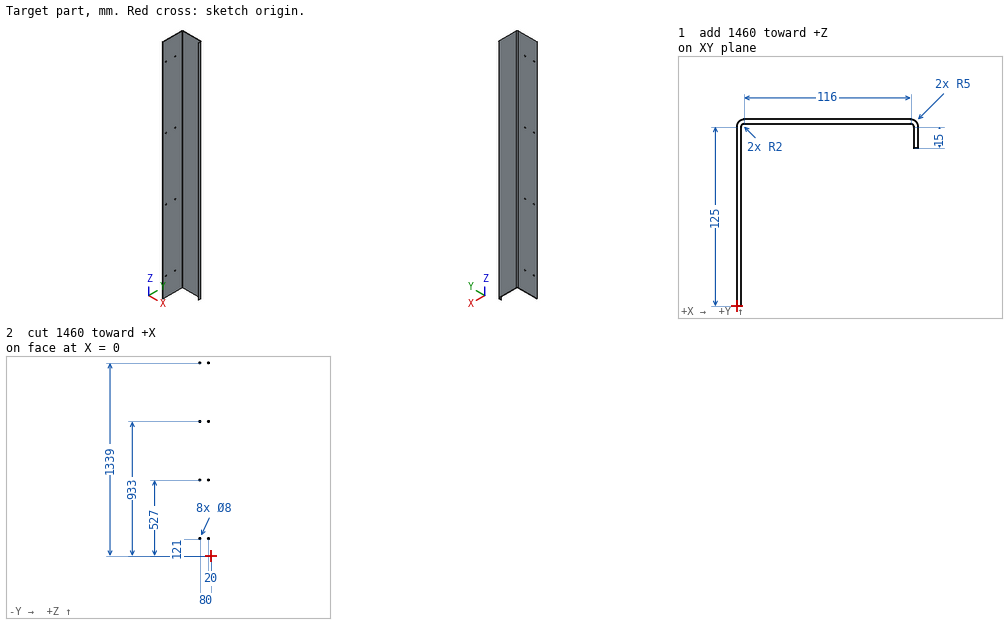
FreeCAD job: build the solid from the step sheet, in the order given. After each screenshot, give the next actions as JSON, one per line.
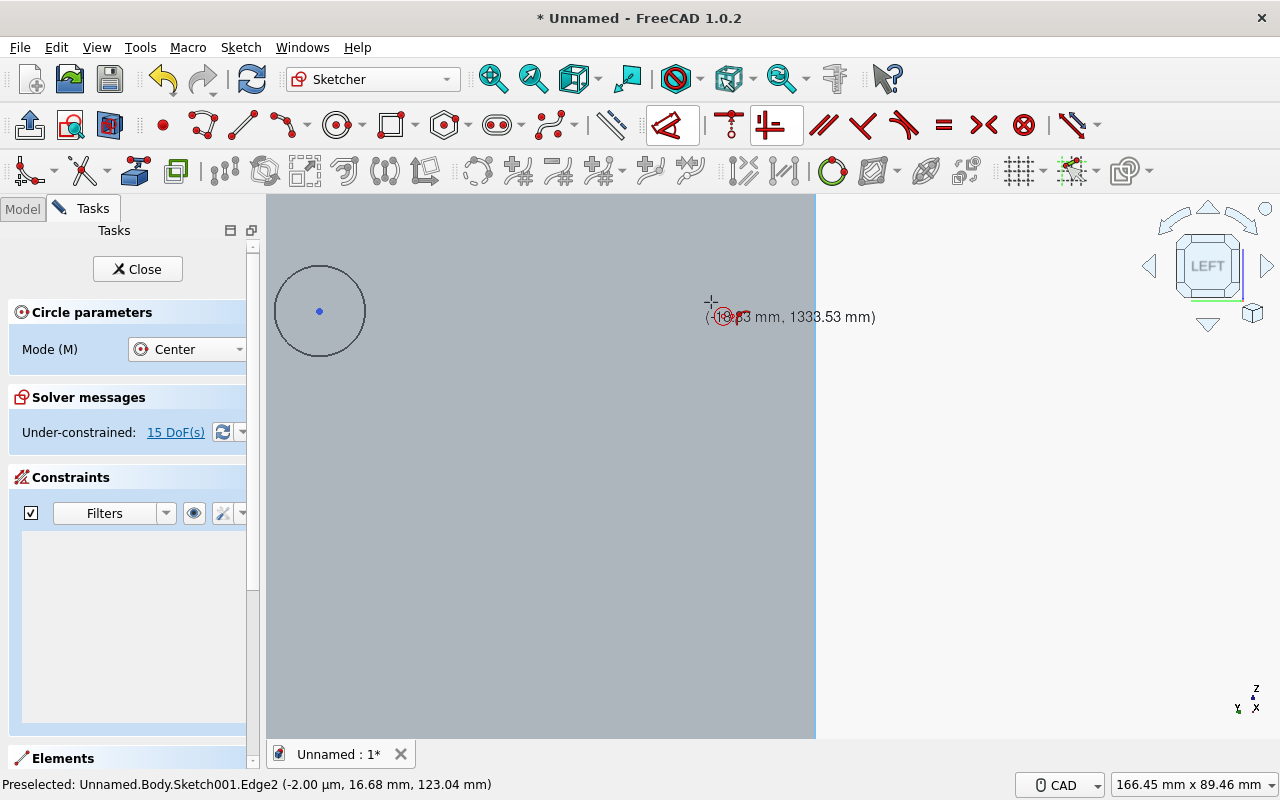
{"action": "scroll", "coordinate": [712, 263], "scroll_direction": "down", "scroll_amount": 15}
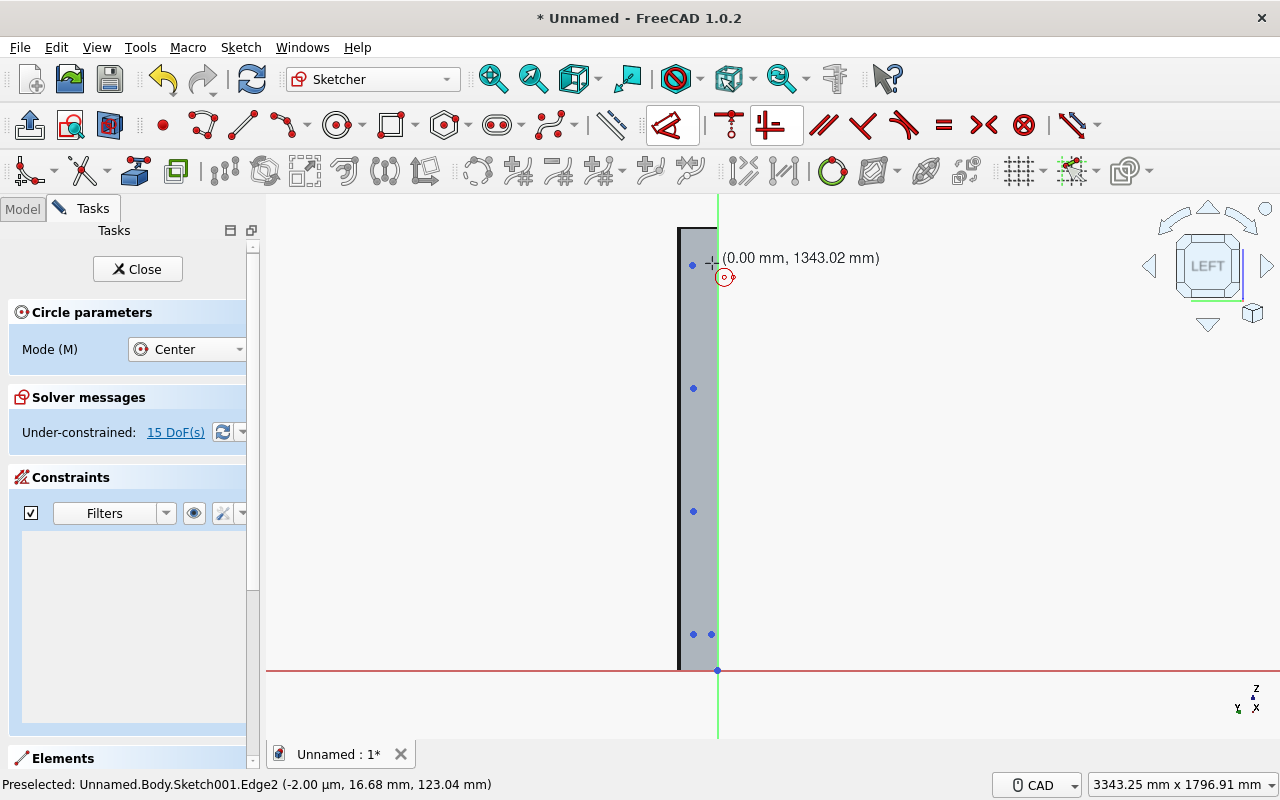
{"action": "scroll", "coordinate": [712, 264], "scroll_direction": "up", "scroll_amount": 5}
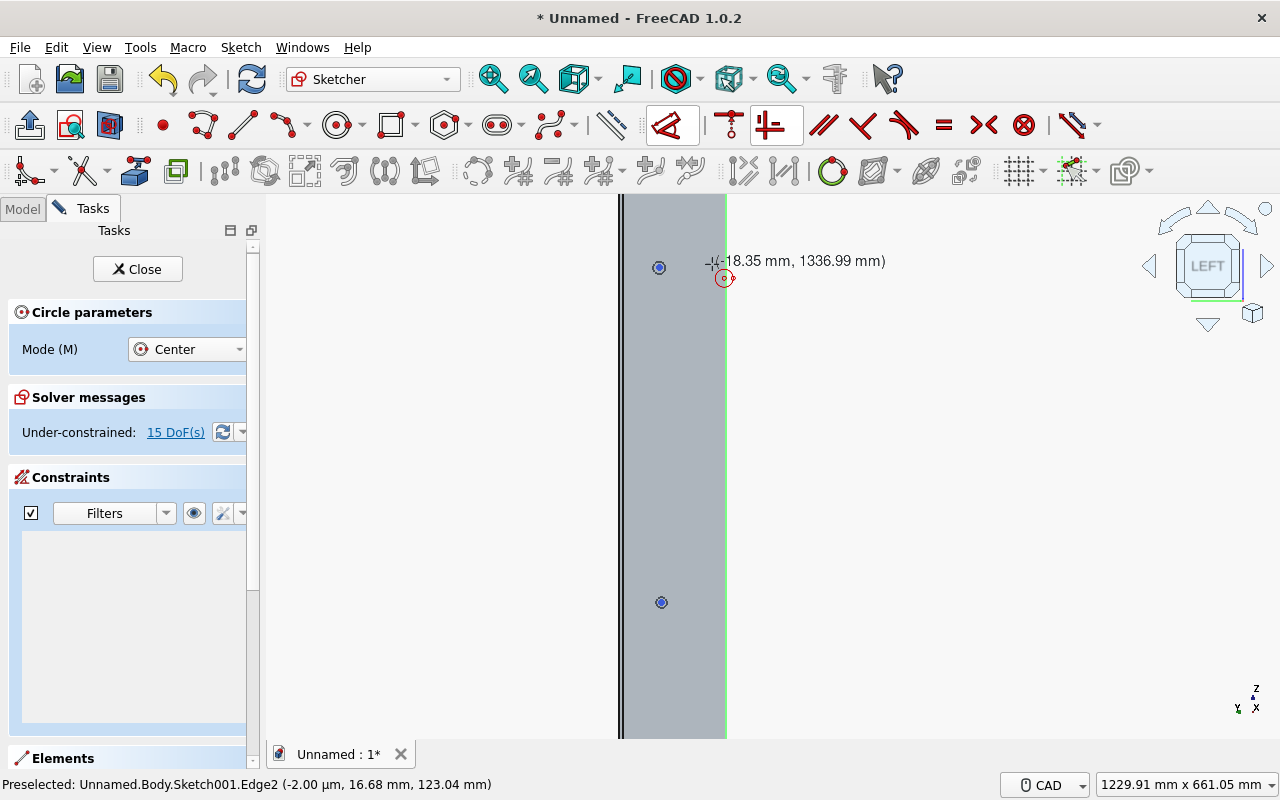
{"action": "left_click", "coordinate": [710, 265]}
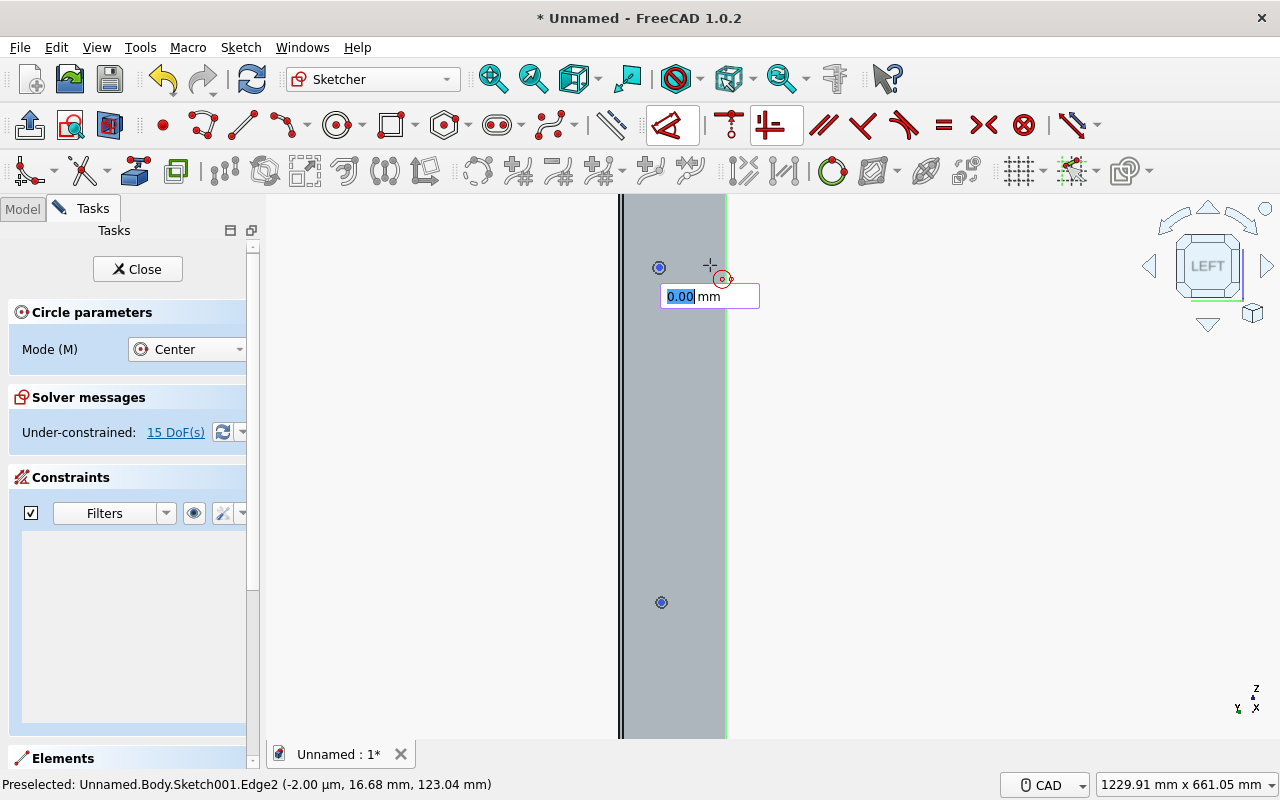
{"action": "scroll", "coordinate": [712, 263], "scroll_direction": "up", "scroll_amount": 8}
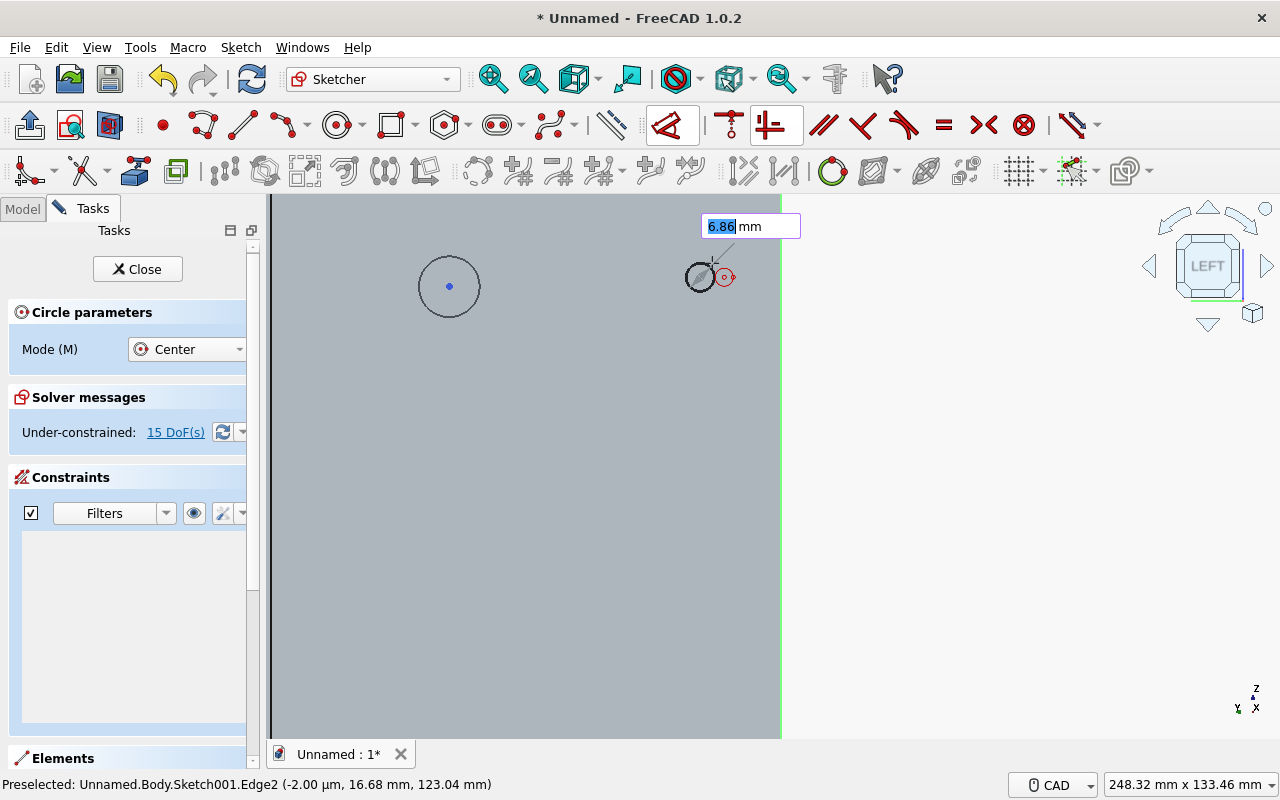
{"action": "left_click", "coordinate": [711, 260]}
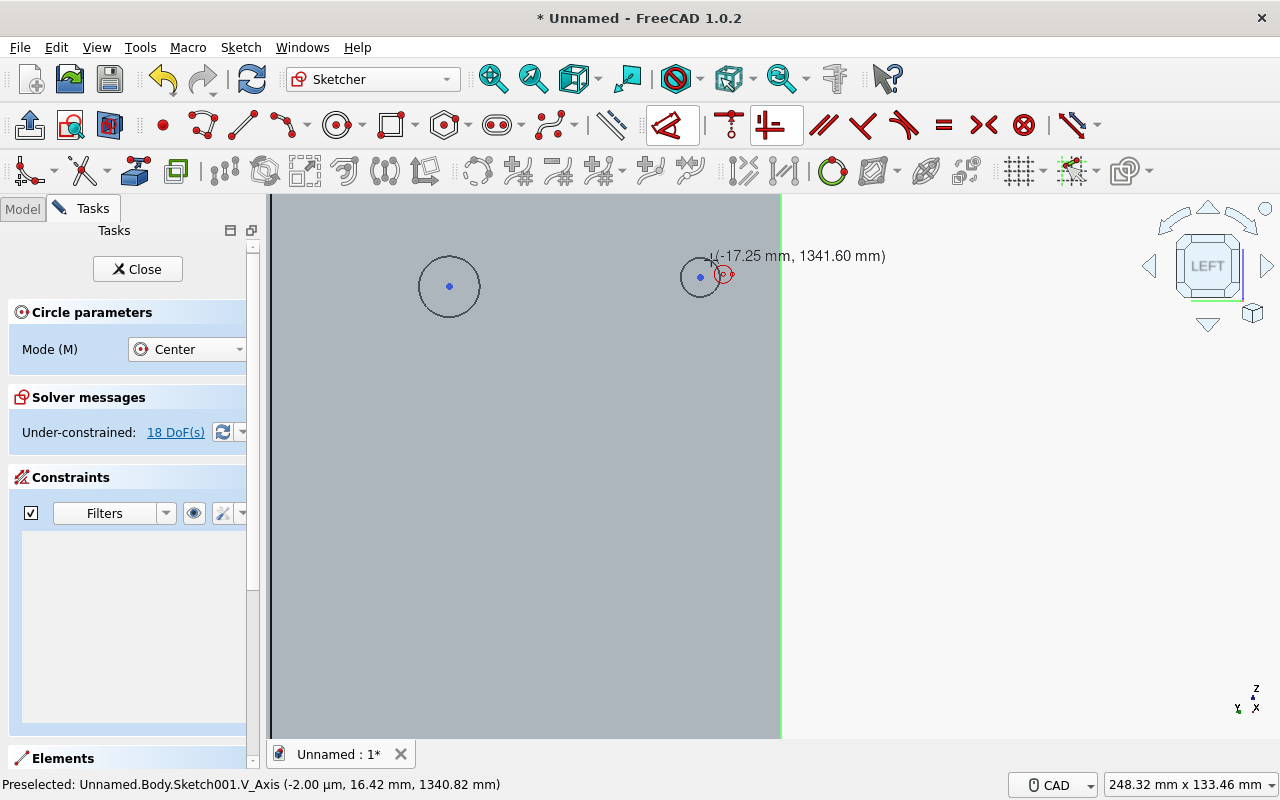
{"action": "scroll", "coordinate": [711, 303], "scroll_direction": "down", "scroll_amount": 14}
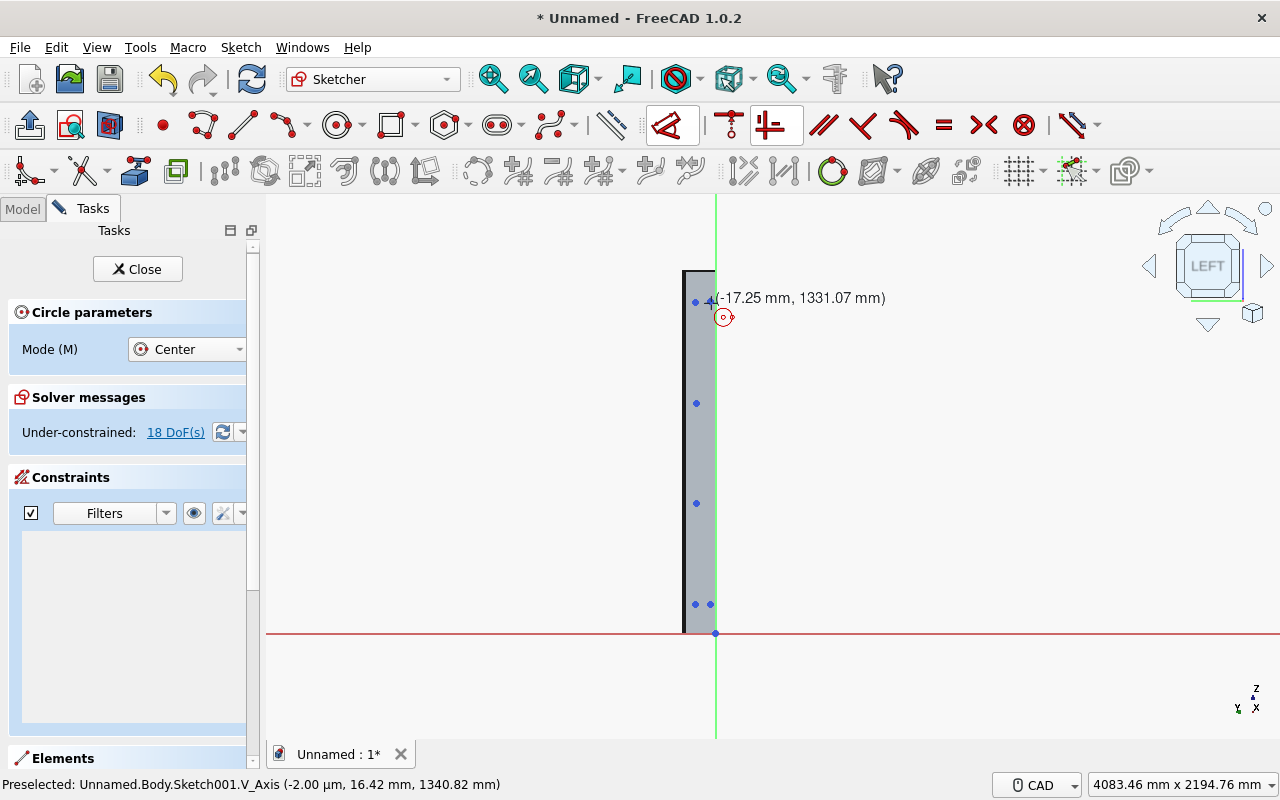
{"action": "scroll", "coordinate": [711, 402], "scroll_direction": "up", "scroll_amount": 16}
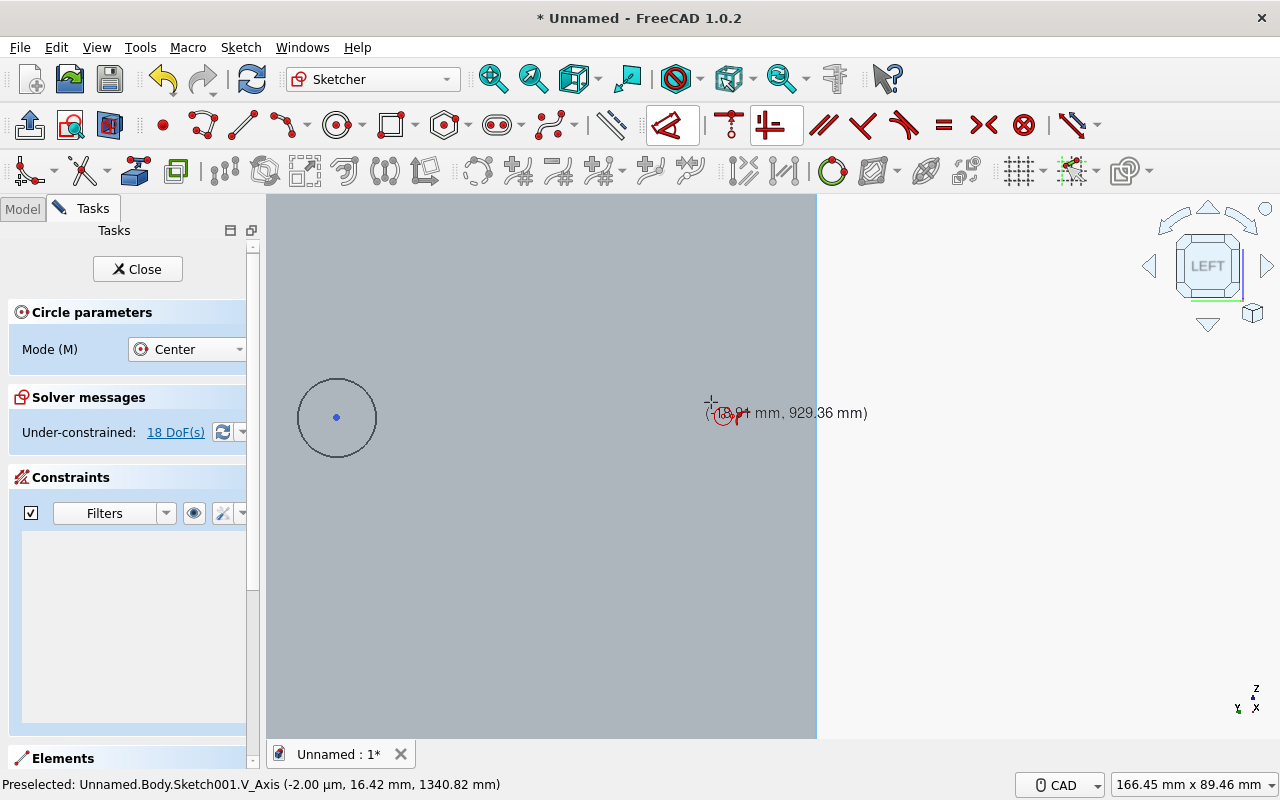
{"action": "scroll", "coordinate": [712, 387], "scroll_direction": "down", "scroll_amount": 15}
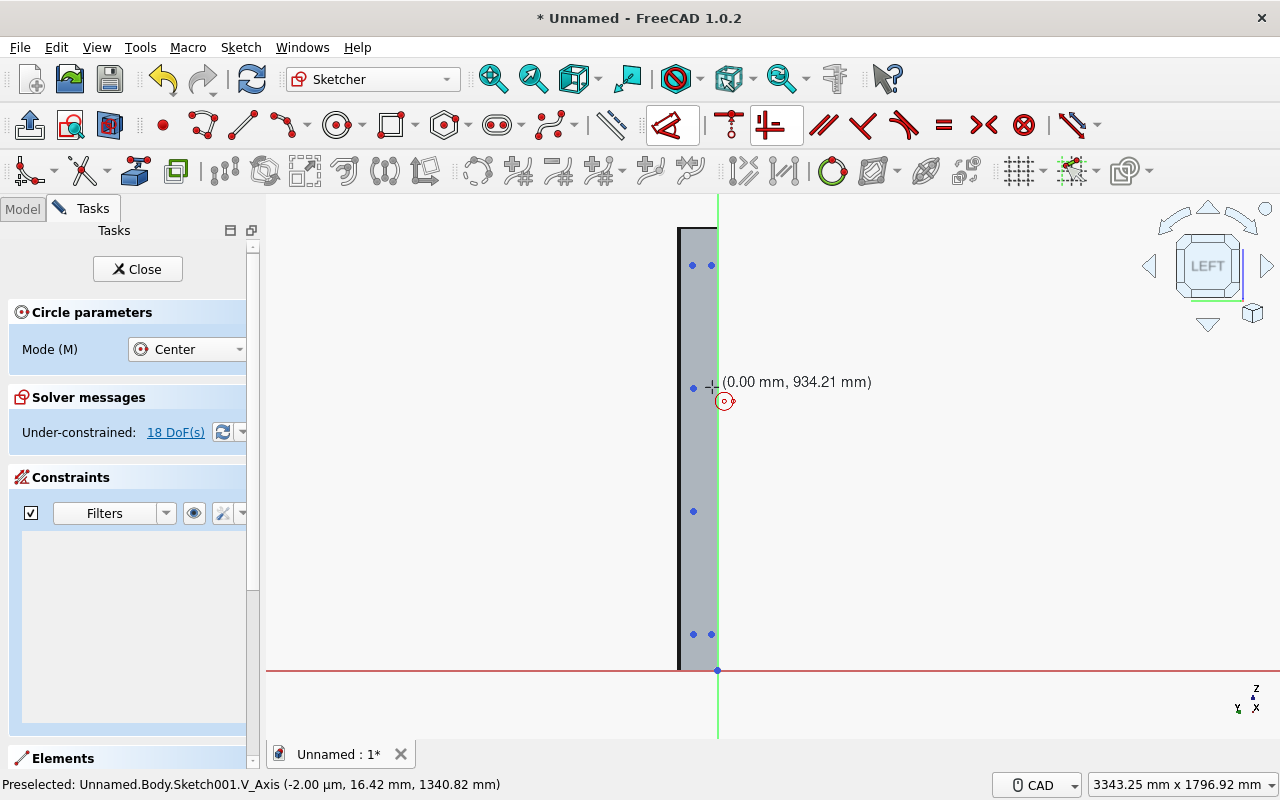
{"action": "scroll", "coordinate": [712, 388], "scroll_direction": "up", "scroll_amount": 5}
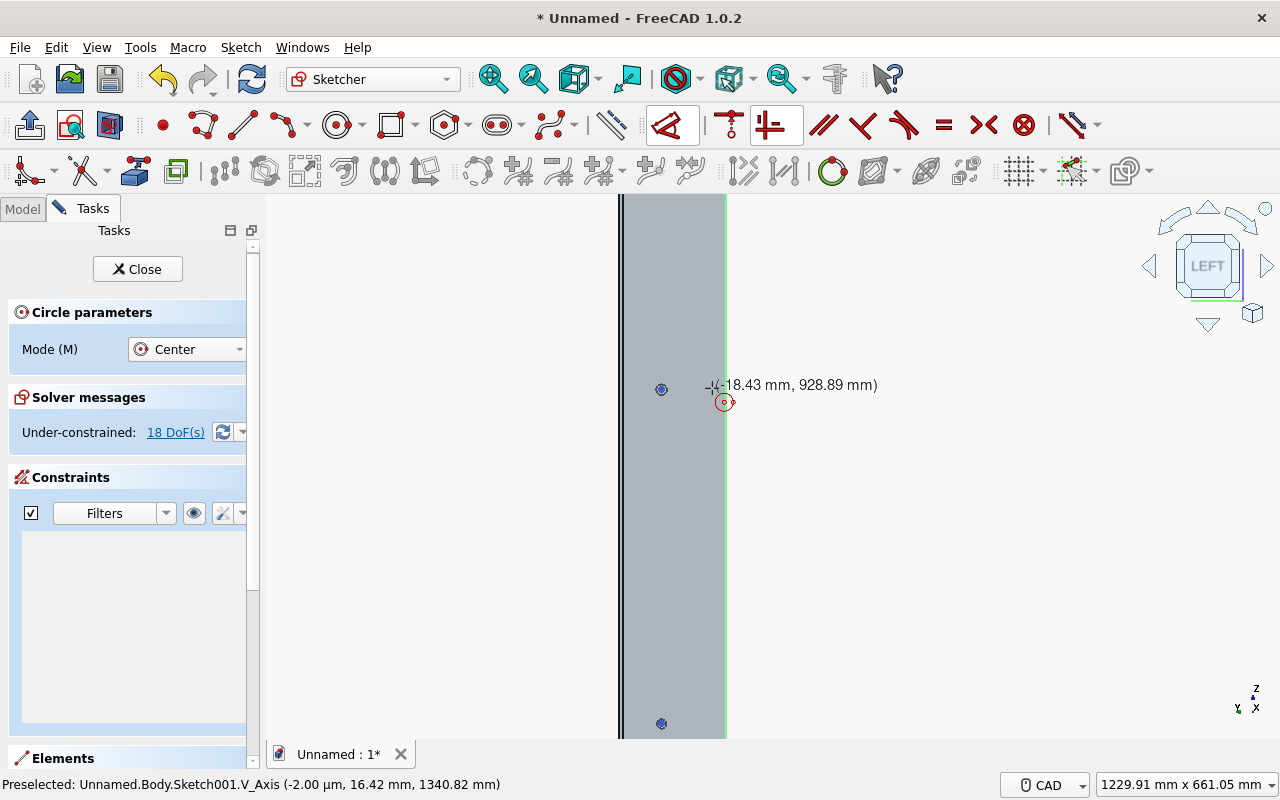
{"action": "left_click", "coordinate": [710, 387]}